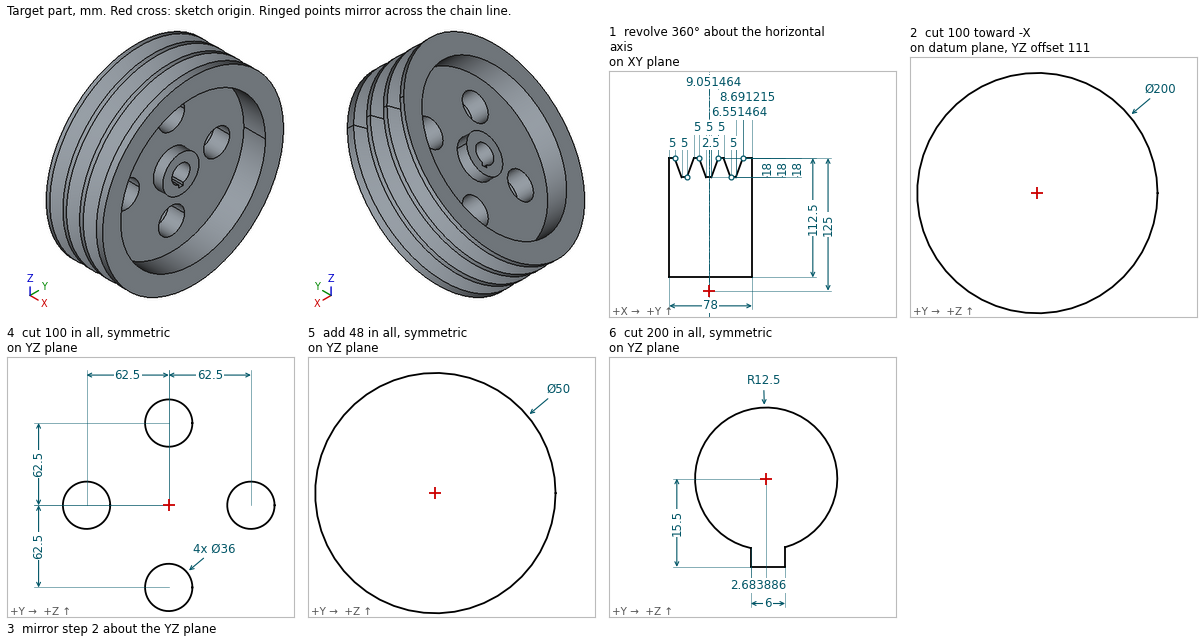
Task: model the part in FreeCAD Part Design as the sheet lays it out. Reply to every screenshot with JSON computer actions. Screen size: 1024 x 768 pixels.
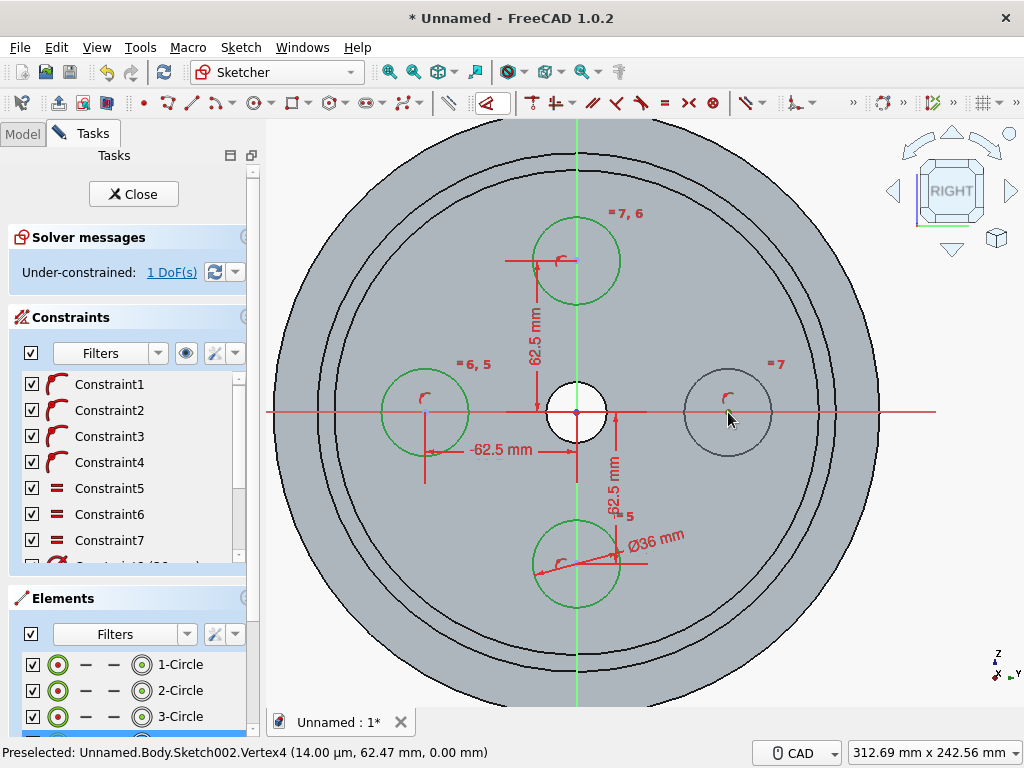
{"action": "left_click", "coordinate": [504, 104]}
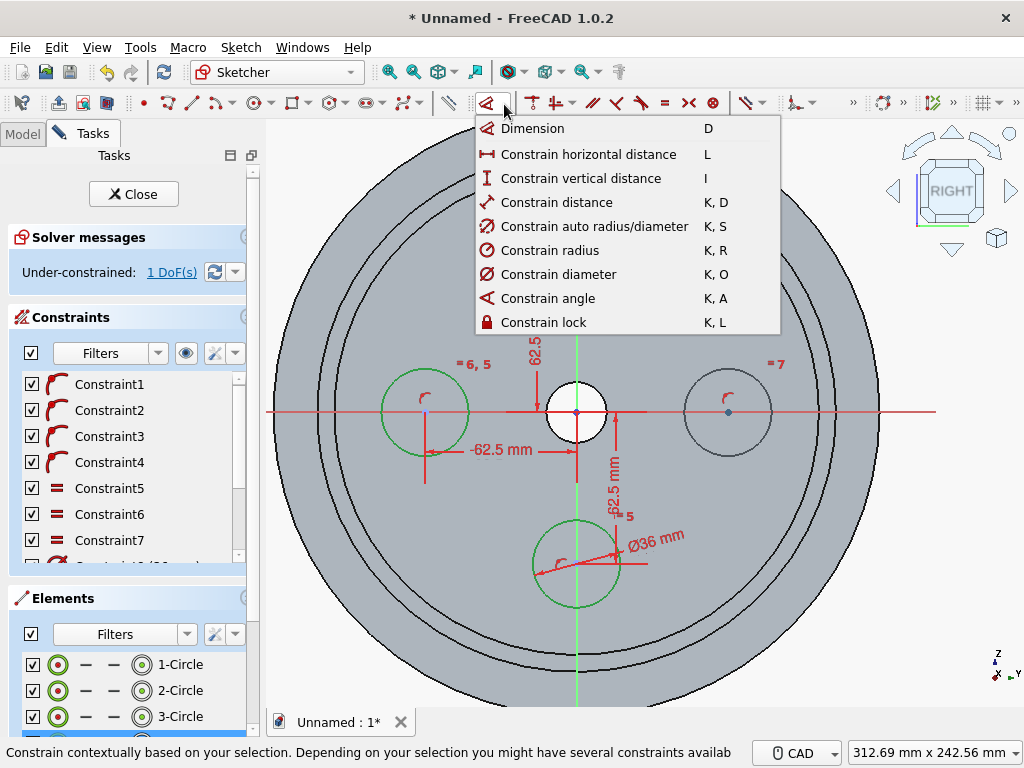
{"action": "left_click", "coordinate": [628, 154]}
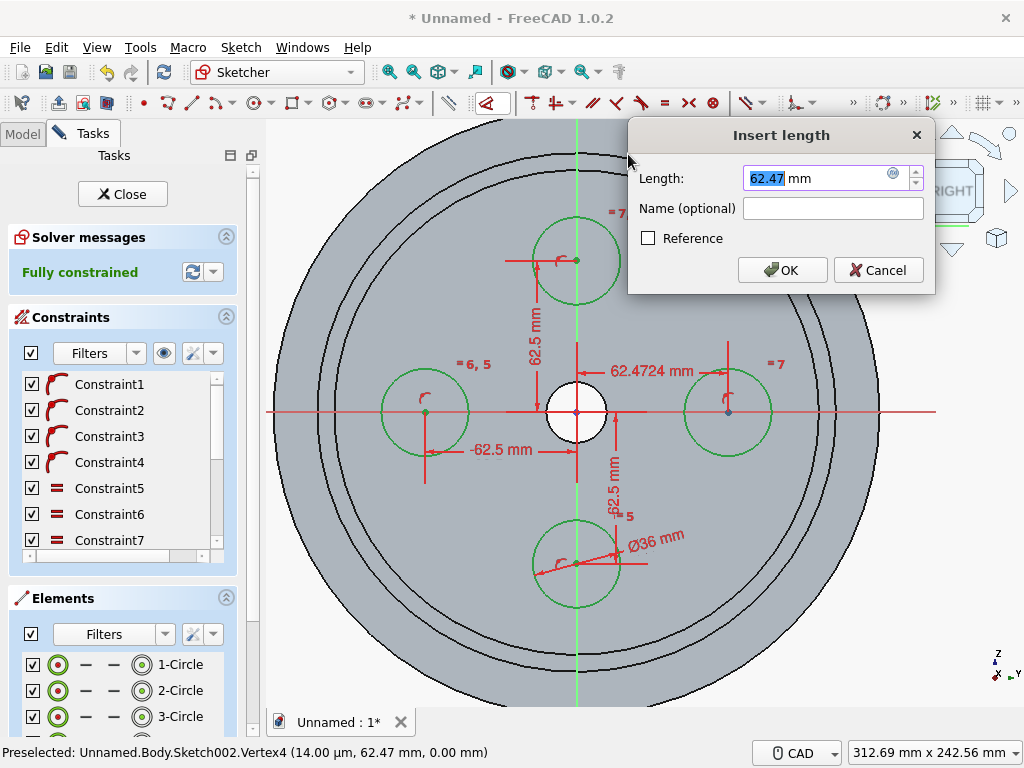
{"action": "type", "text": "62.5"}
{"action": "key", "text": "Return"}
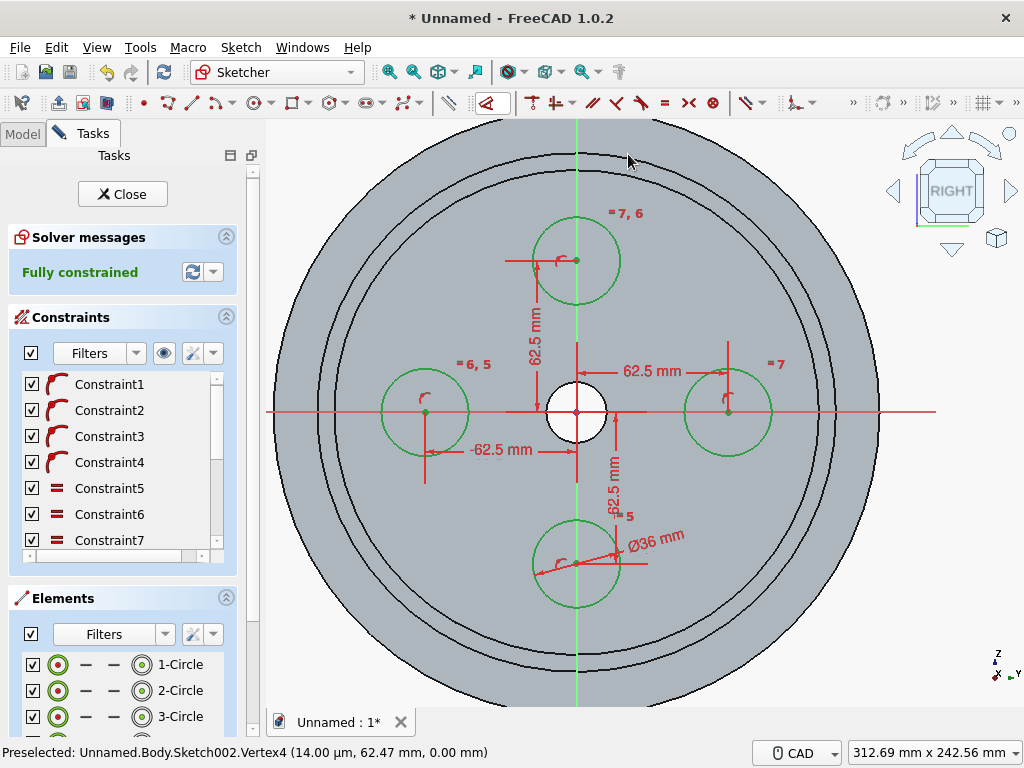
{"action": "left_click", "coordinate": [123, 194]}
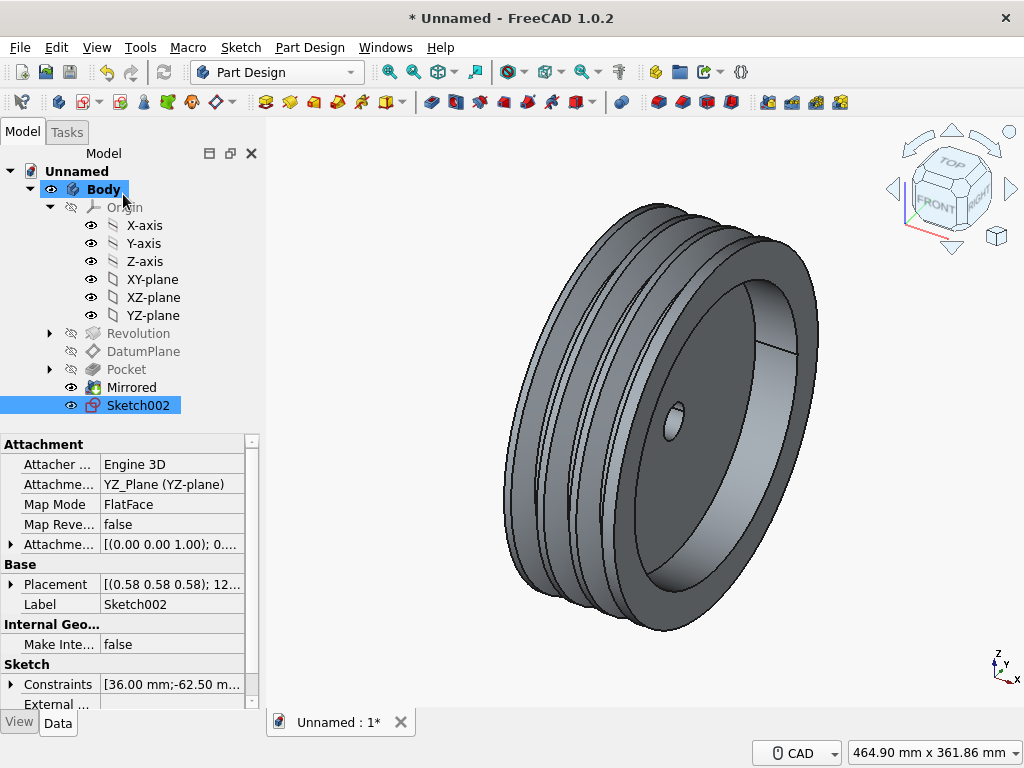
{"action": "left_click", "coordinate": [432, 102]}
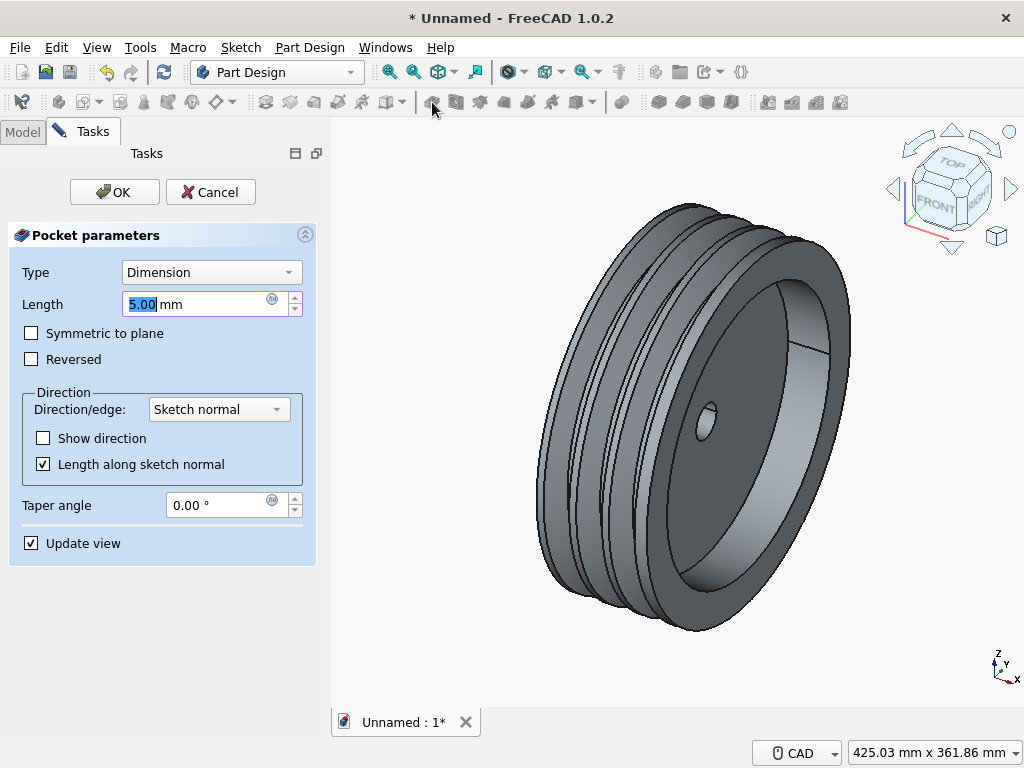
{"action": "type", "text": "100"}
{"action": "key", "text": "Tab"}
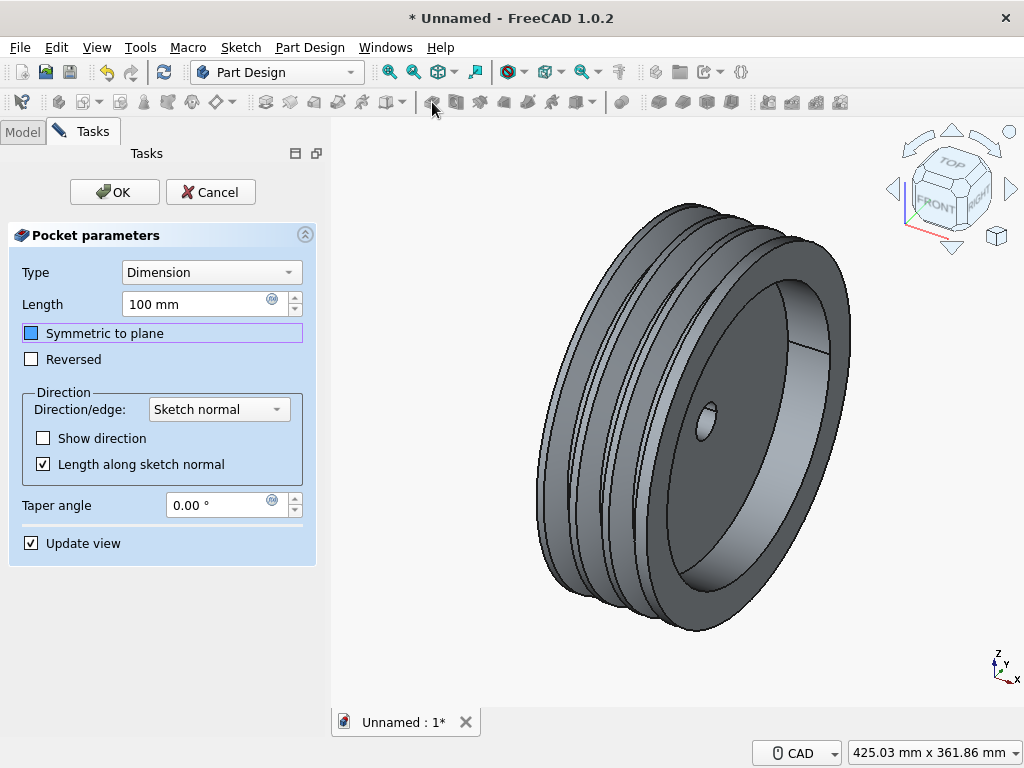
{"action": "left_click", "coordinate": [30, 333]}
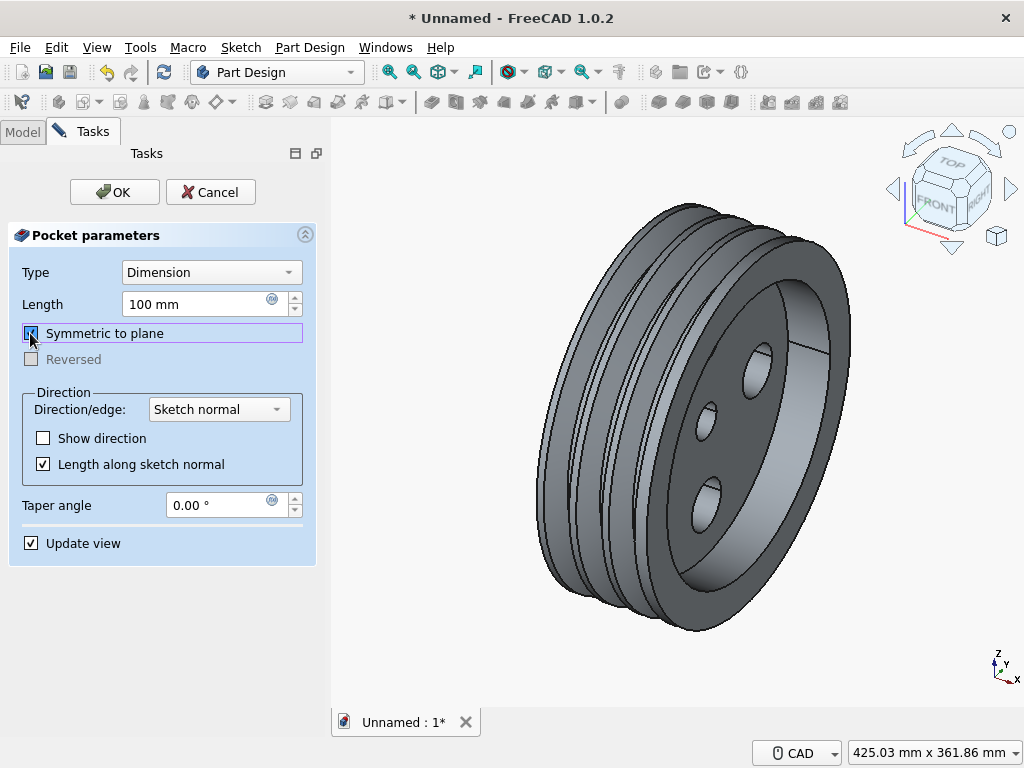
{"action": "left_click", "coordinate": [115, 192]}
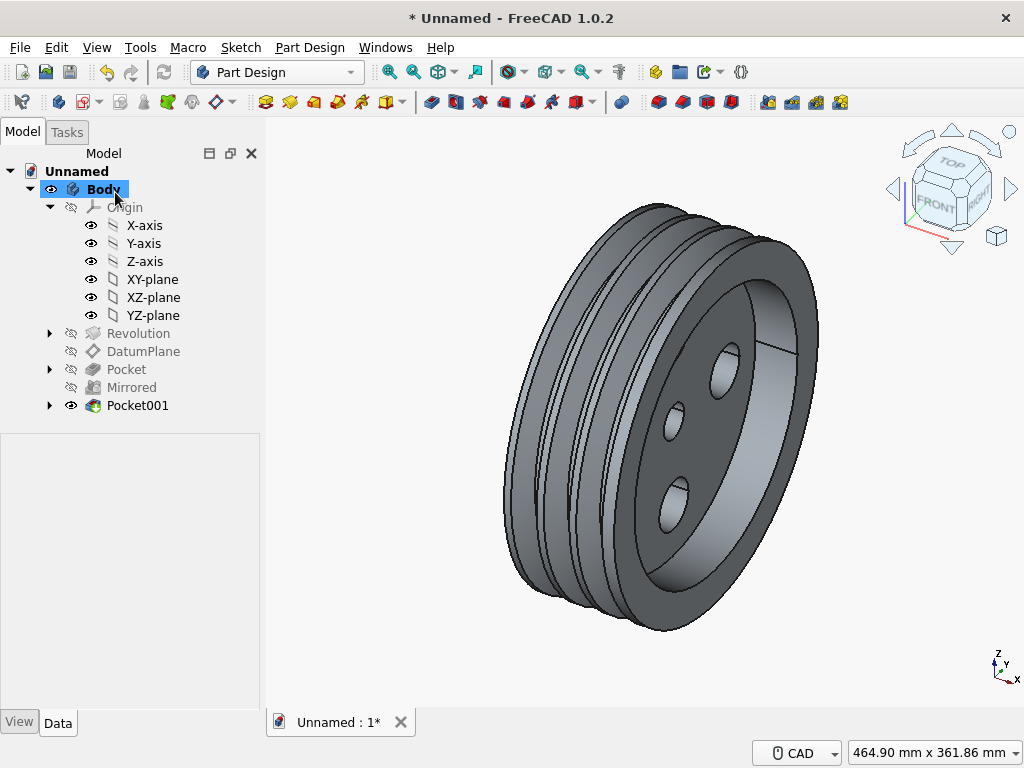
{"action": "left_click", "coordinate": [84, 102]}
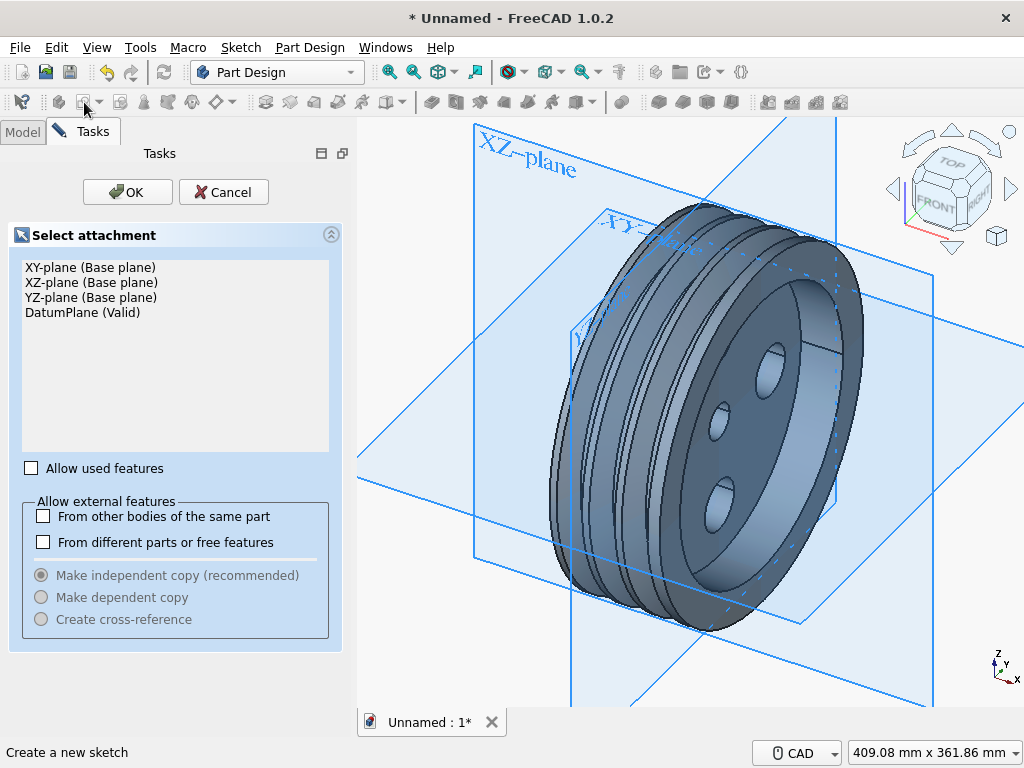
{"action": "left_click", "coordinate": [82, 298]}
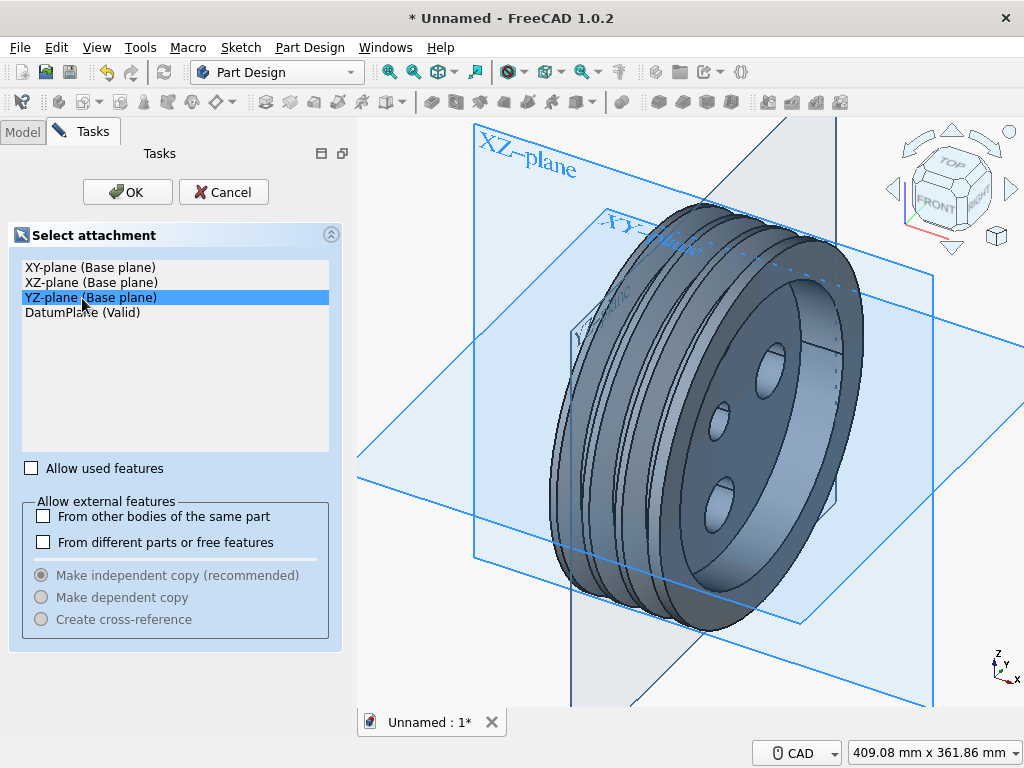
{"action": "left_click", "coordinate": [128, 192]}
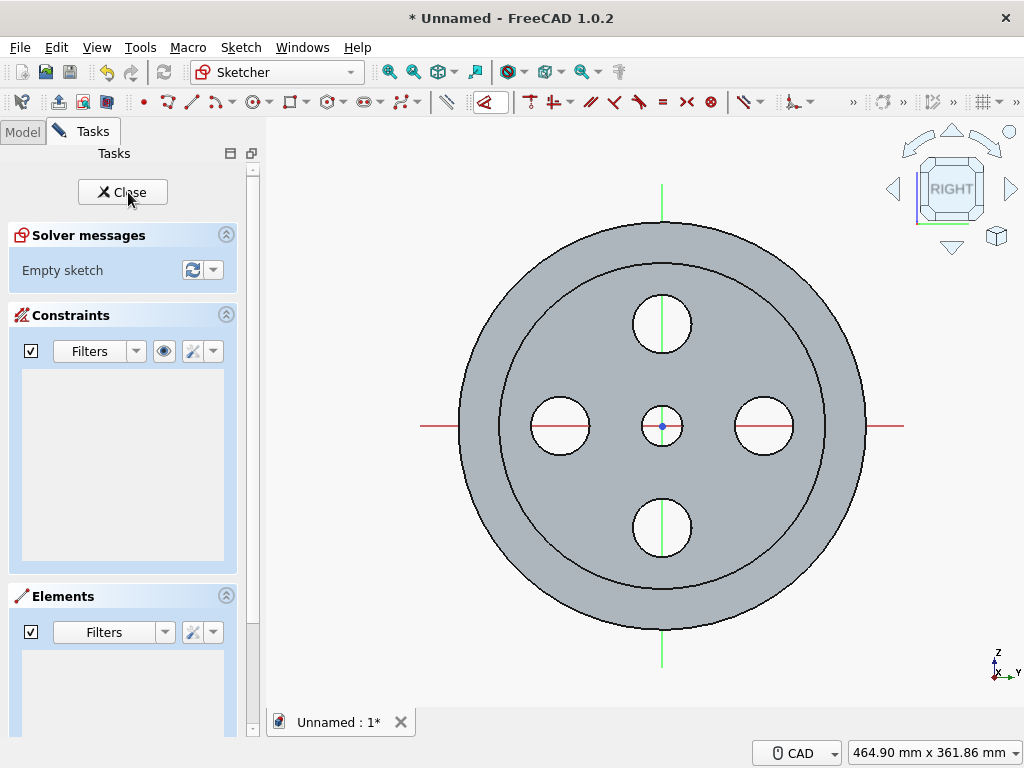
{"action": "left_click", "coordinate": [108, 102]}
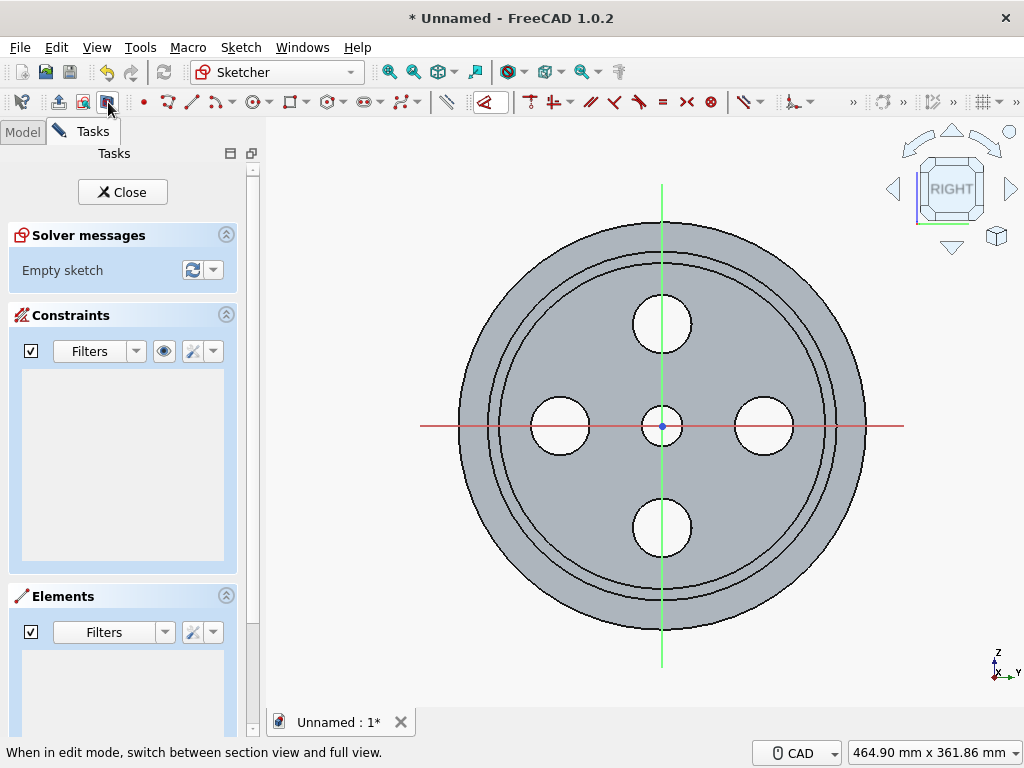
{"action": "scroll", "coordinate": [684, 430], "scroll_direction": "up", "scroll_amount": 8}